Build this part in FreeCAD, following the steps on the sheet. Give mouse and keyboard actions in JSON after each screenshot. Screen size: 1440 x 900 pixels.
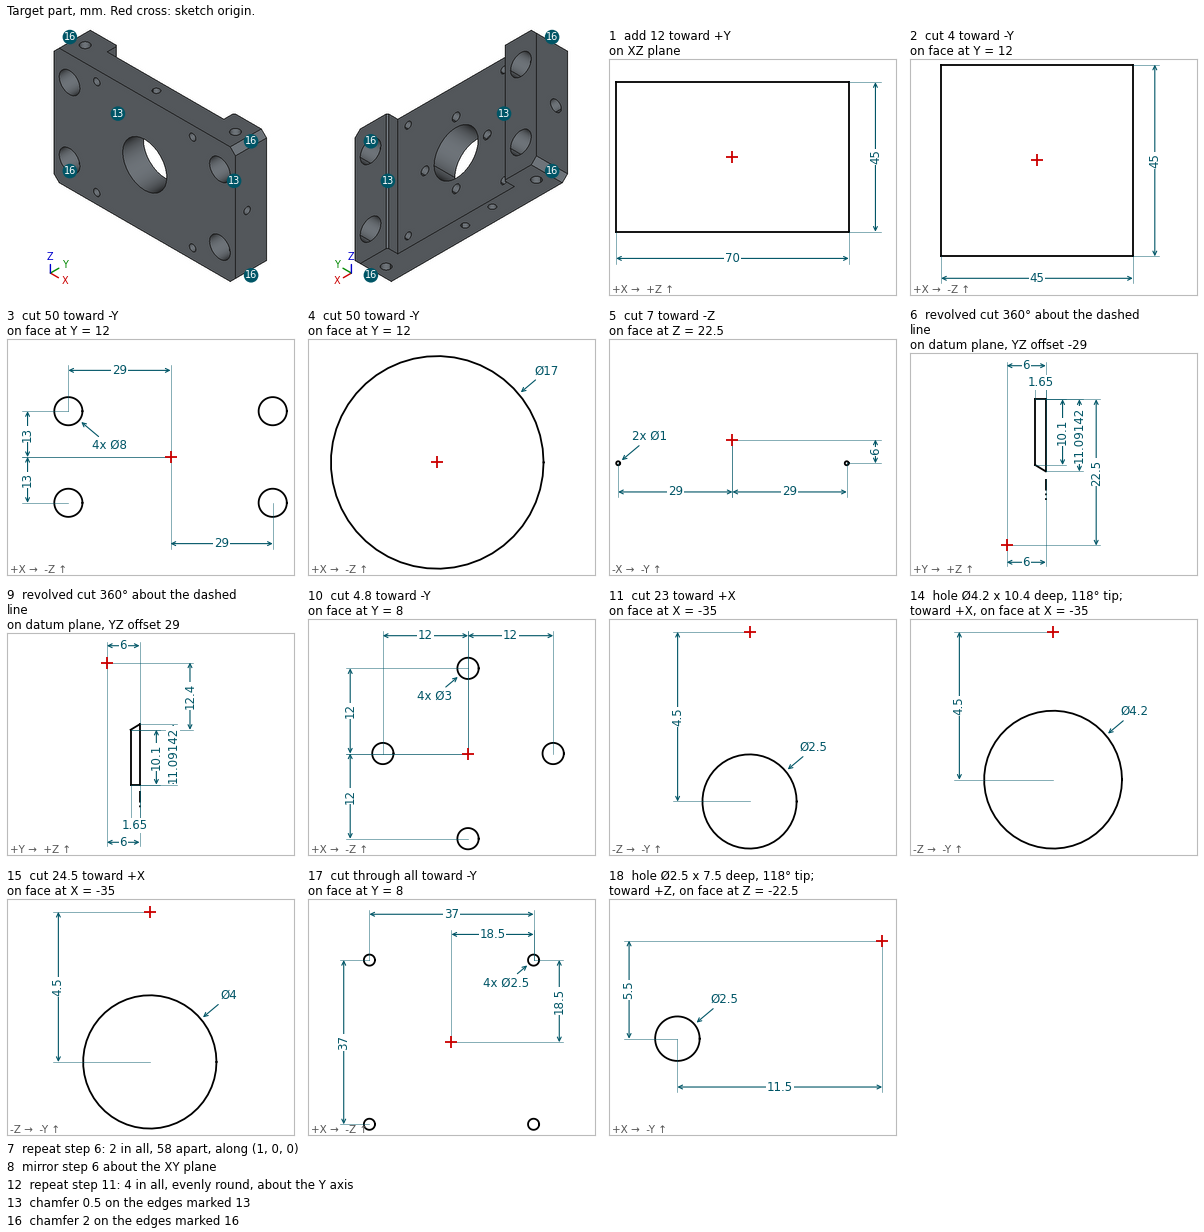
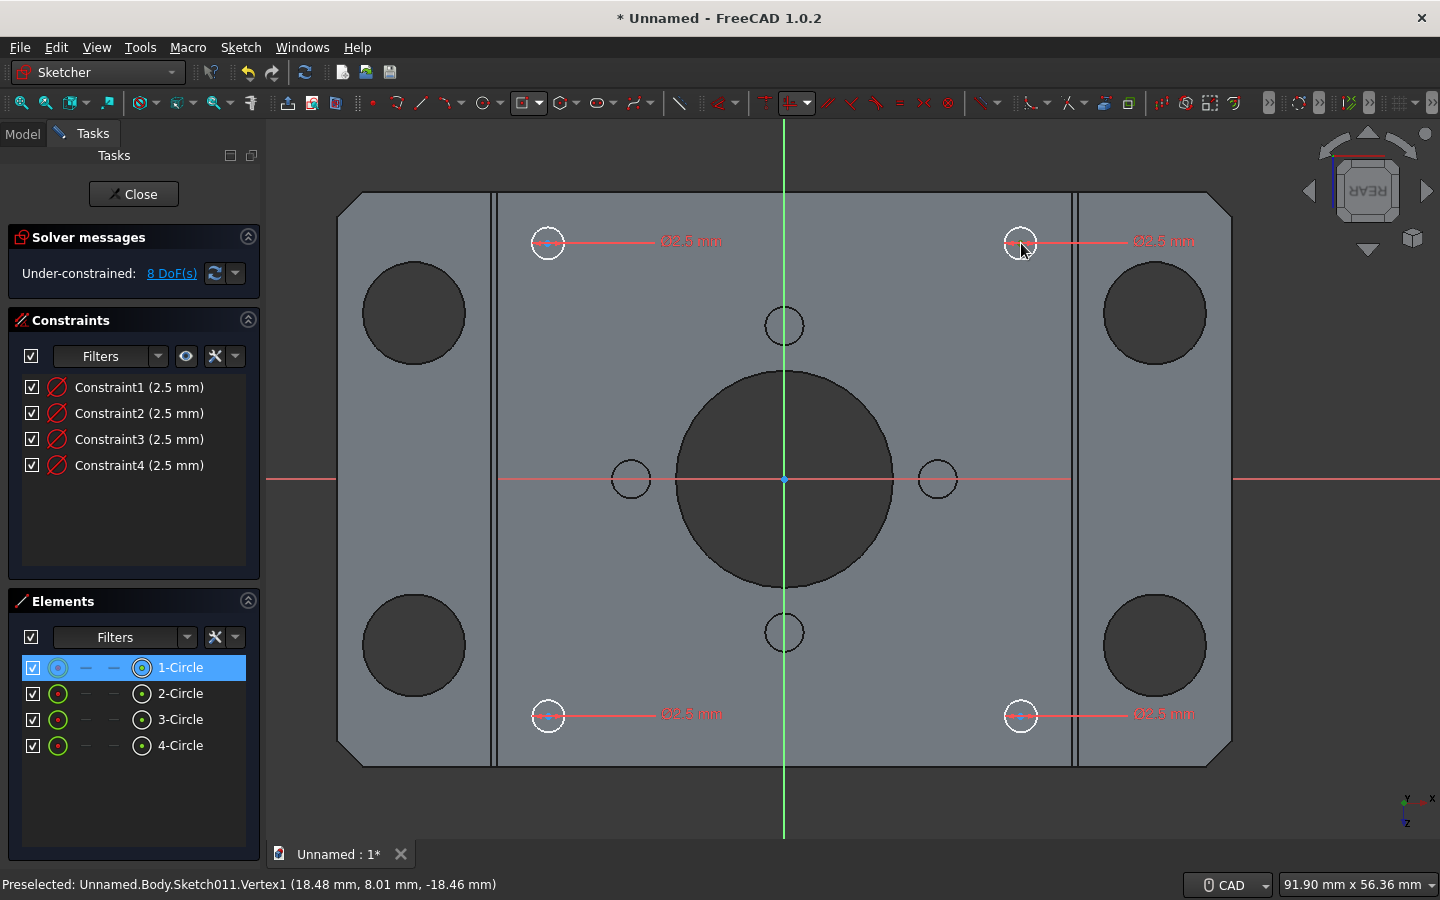
{"action": "left_click", "coordinate": [548, 243]}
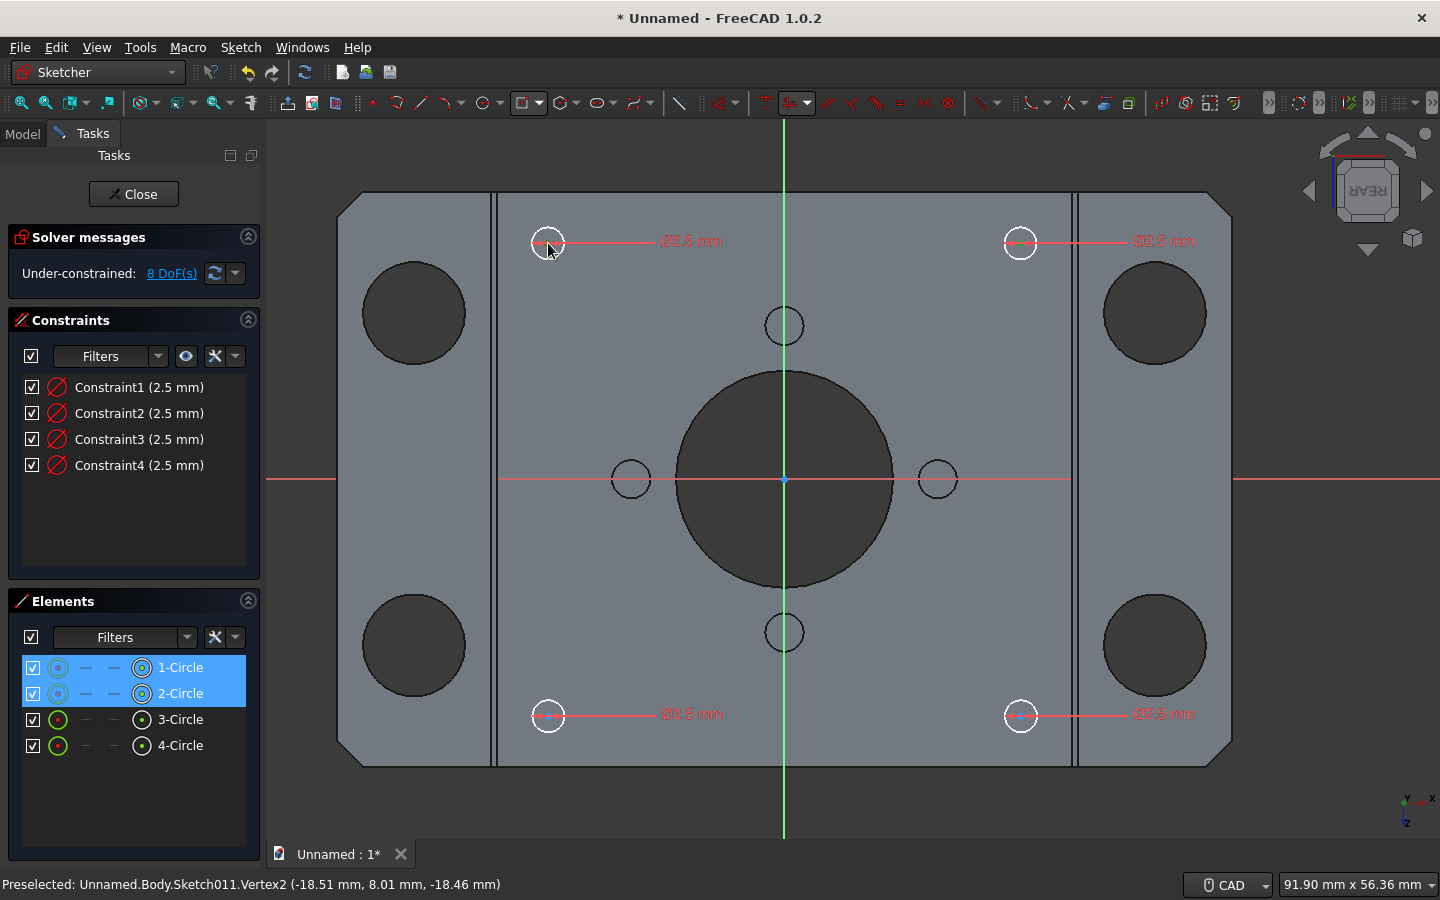
{"action": "key", "text": "h"}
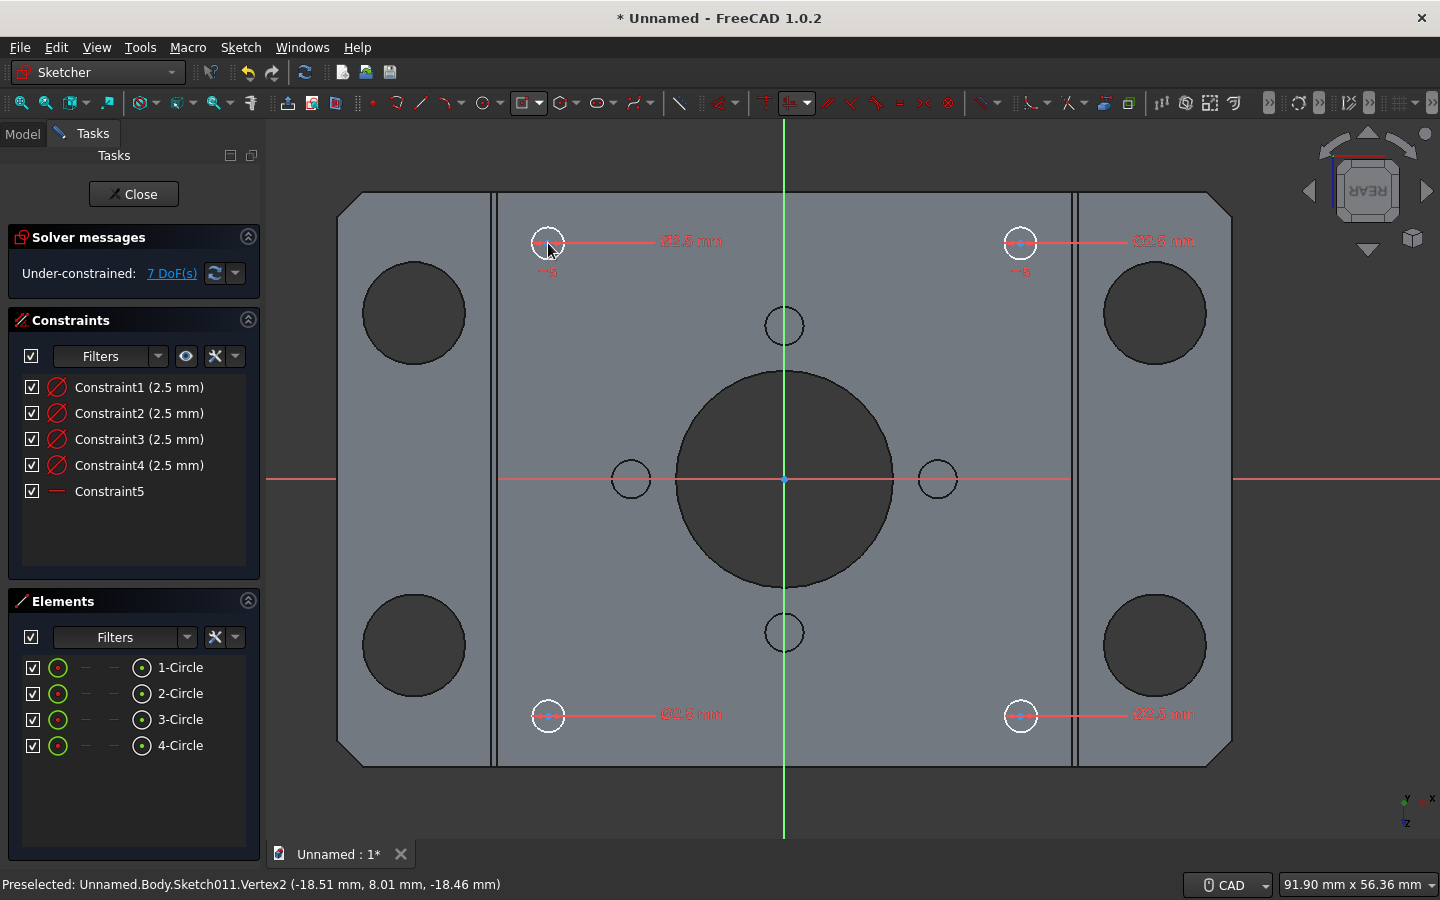
{"action": "left_click", "coordinate": [548, 243]}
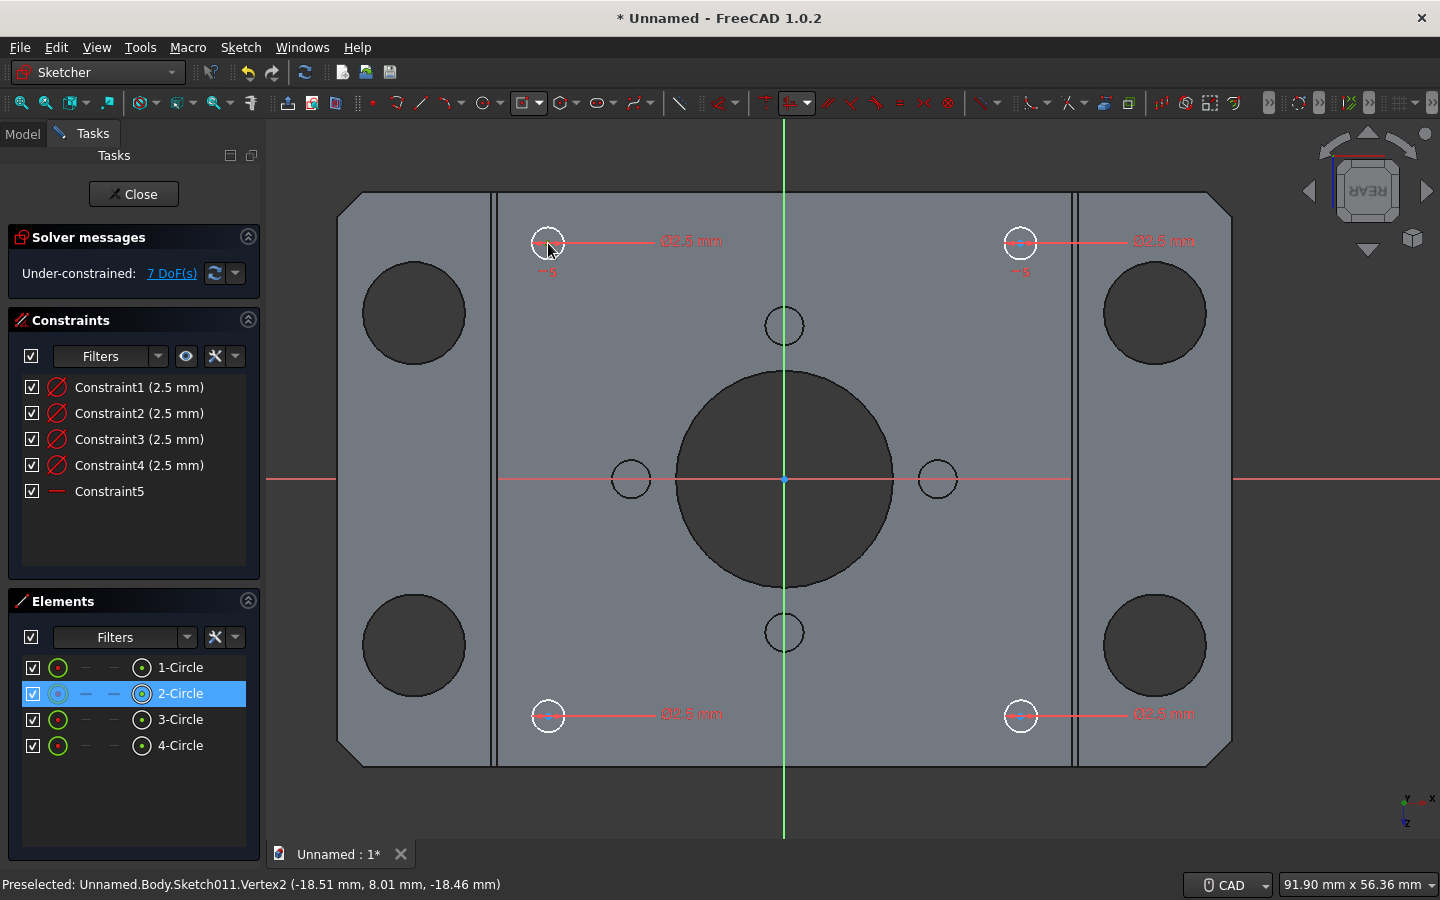
{"action": "left_click", "coordinate": [548, 716]}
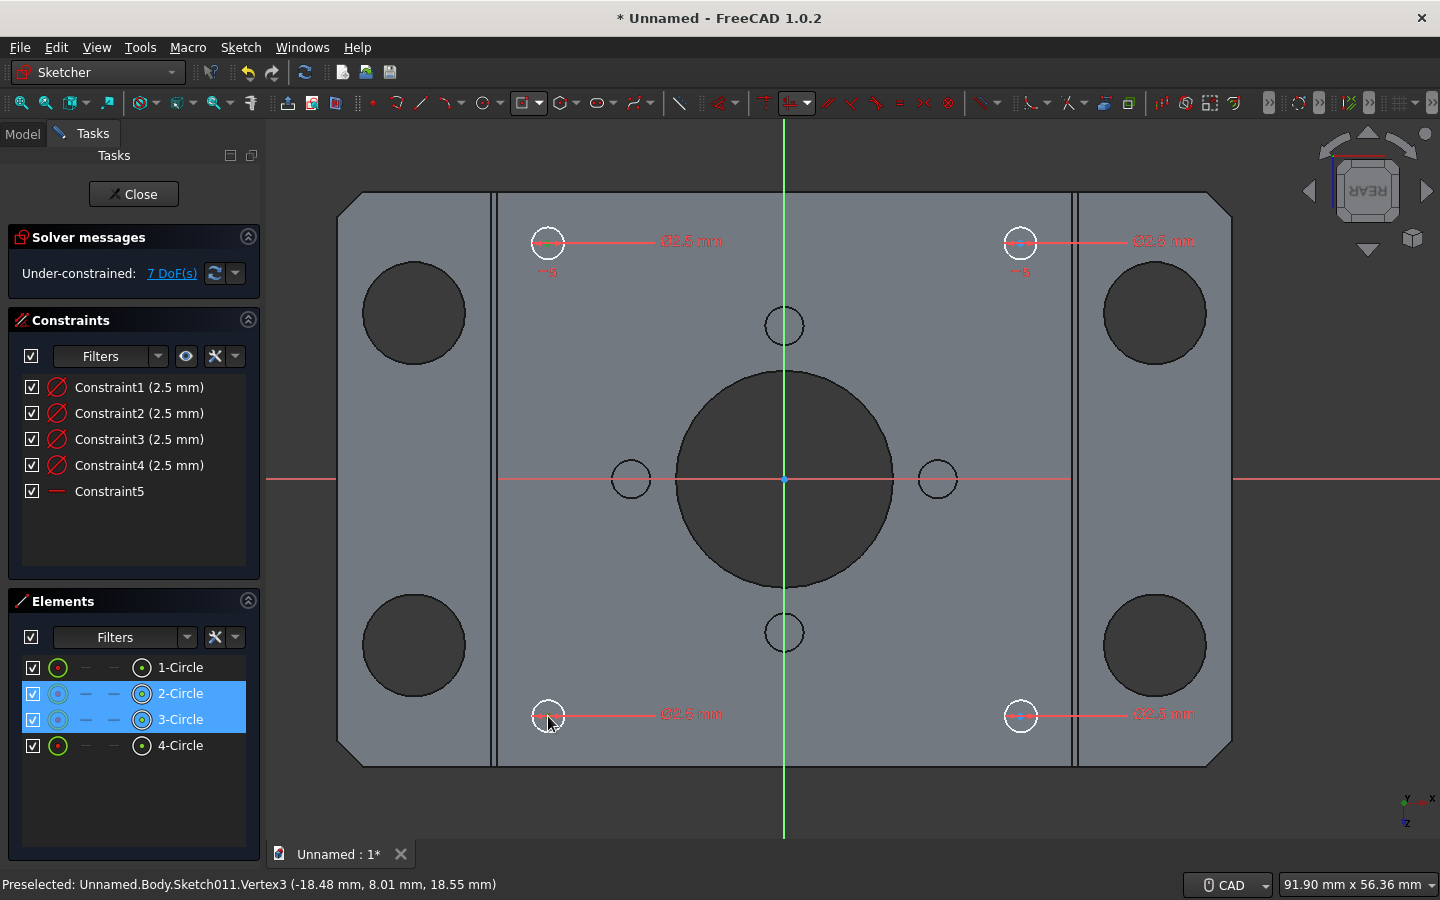
{"action": "left_click", "coordinate": [810, 104]}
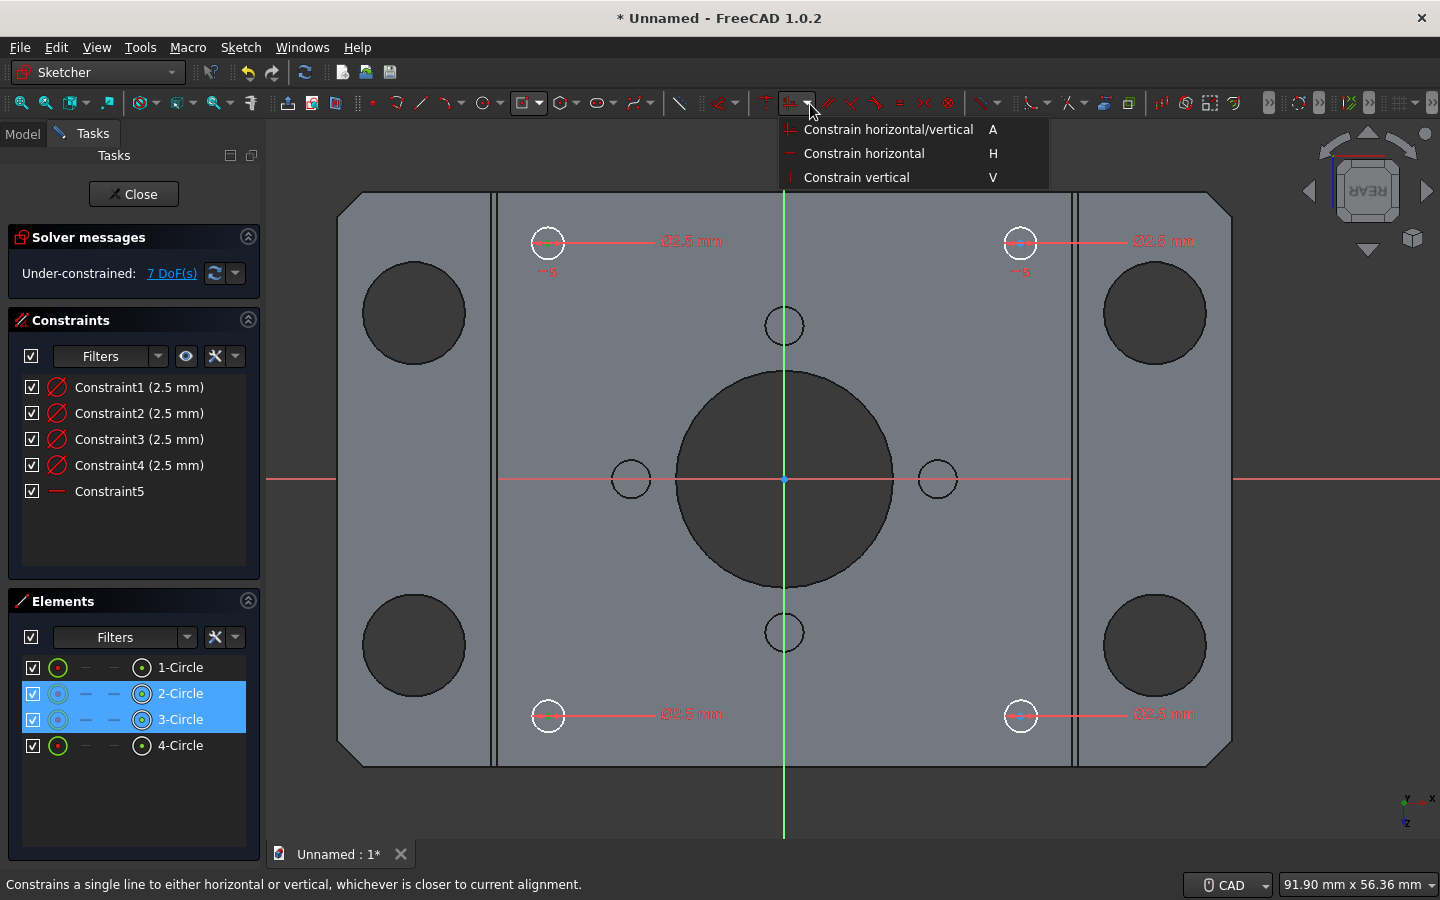
{"action": "left_click", "coordinate": [914, 177]}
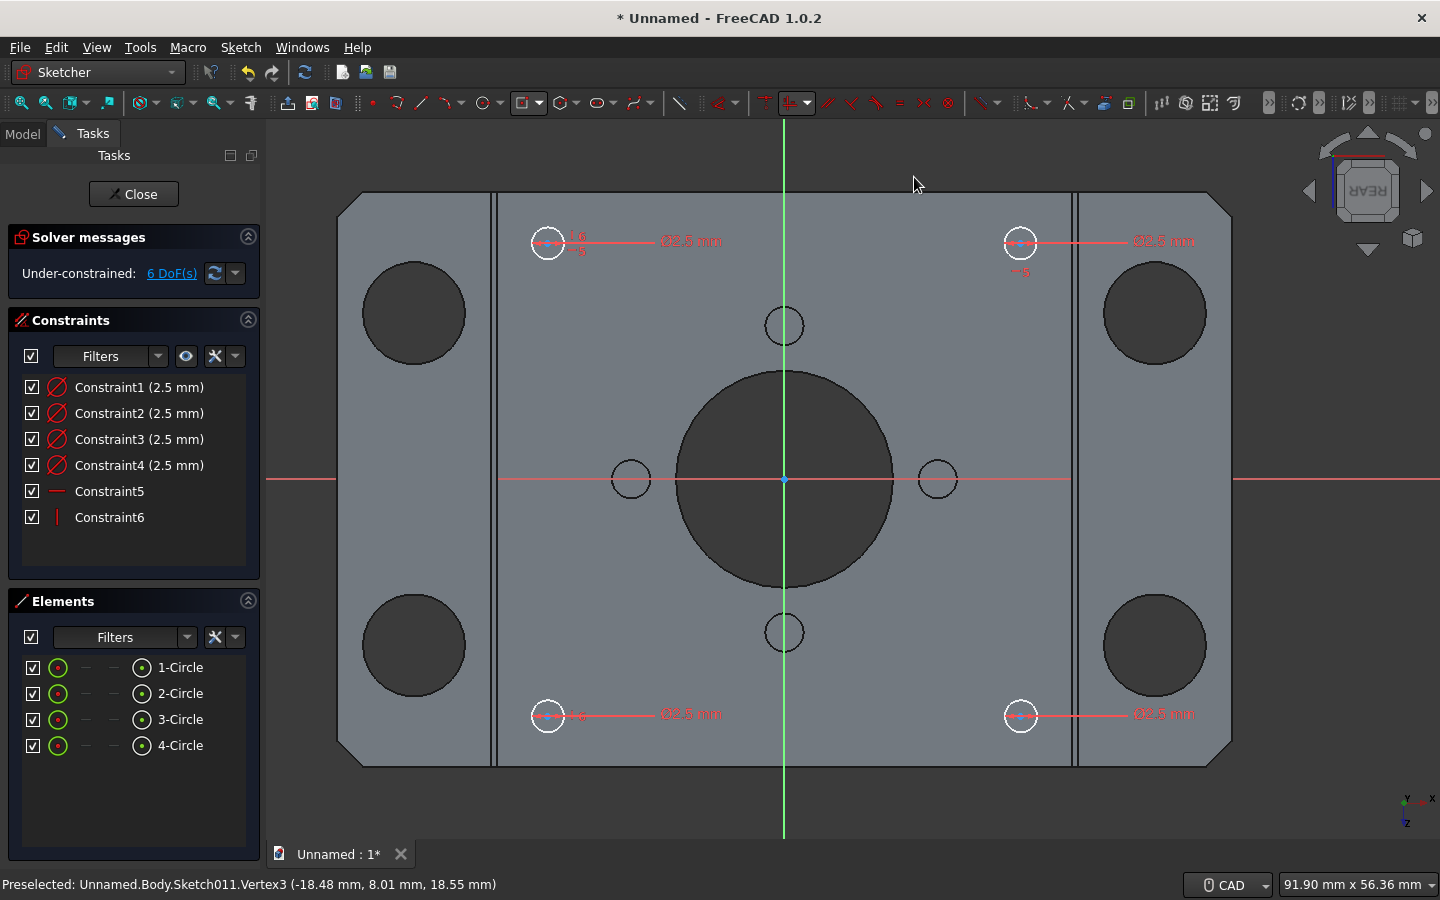
{"action": "left_click", "coordinate": [1021, 243]}